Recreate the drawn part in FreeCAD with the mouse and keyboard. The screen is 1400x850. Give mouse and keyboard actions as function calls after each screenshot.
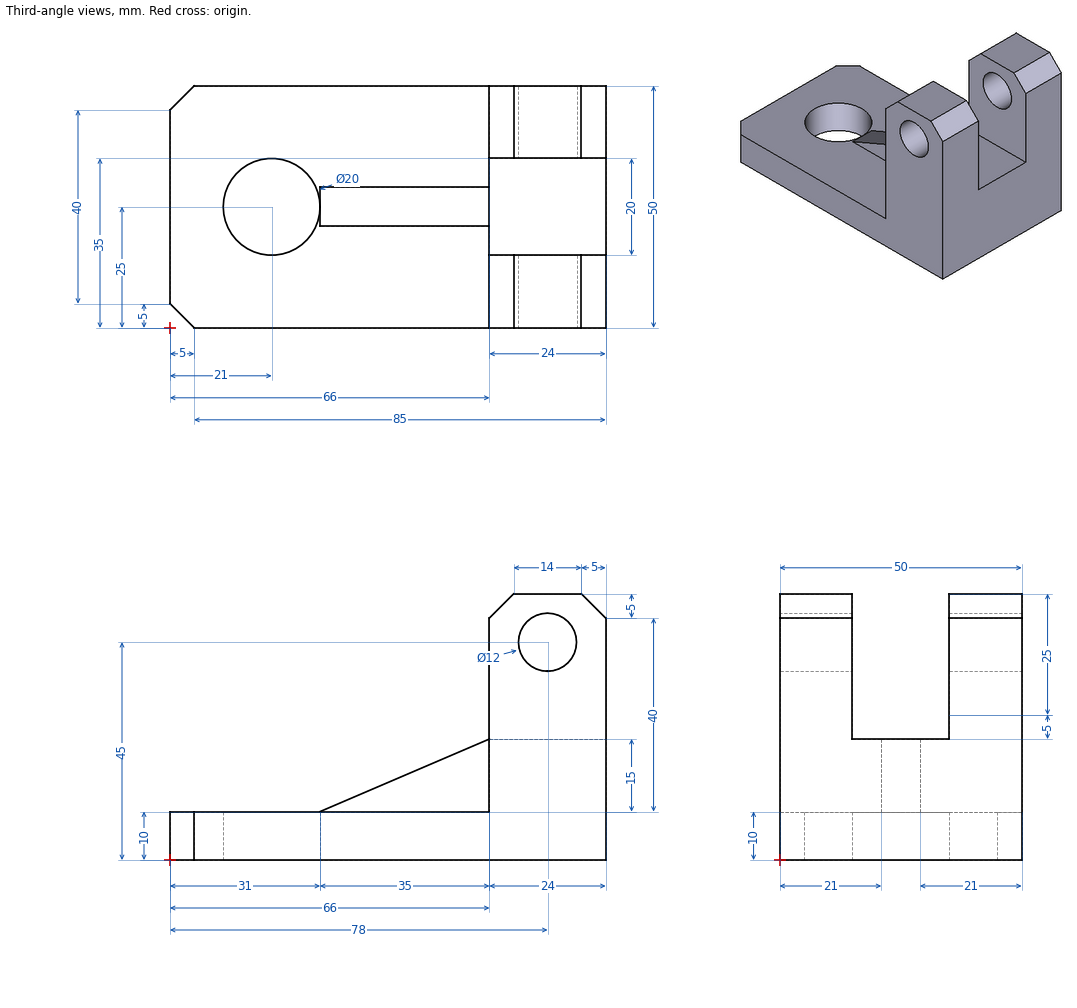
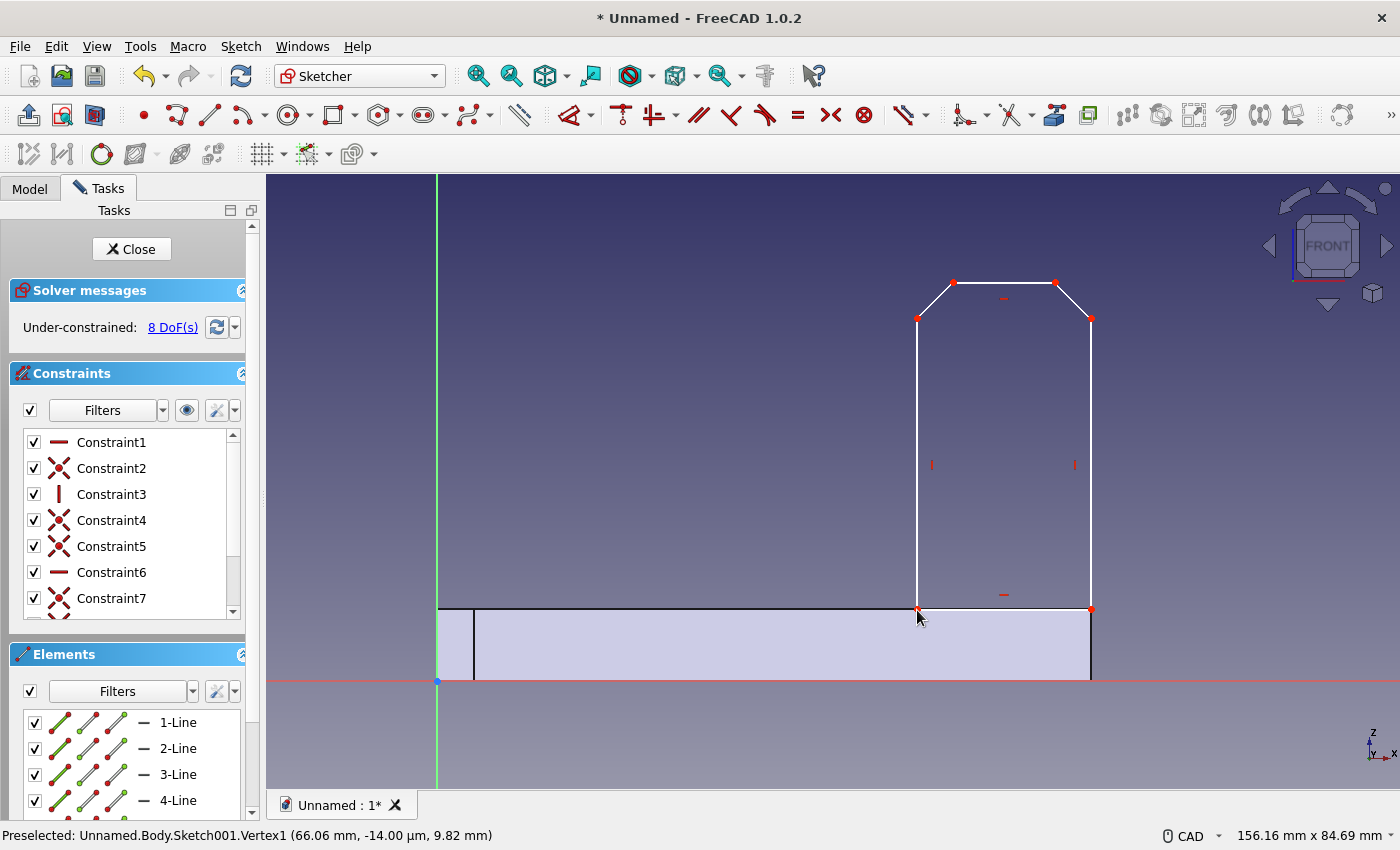
click(568, 116)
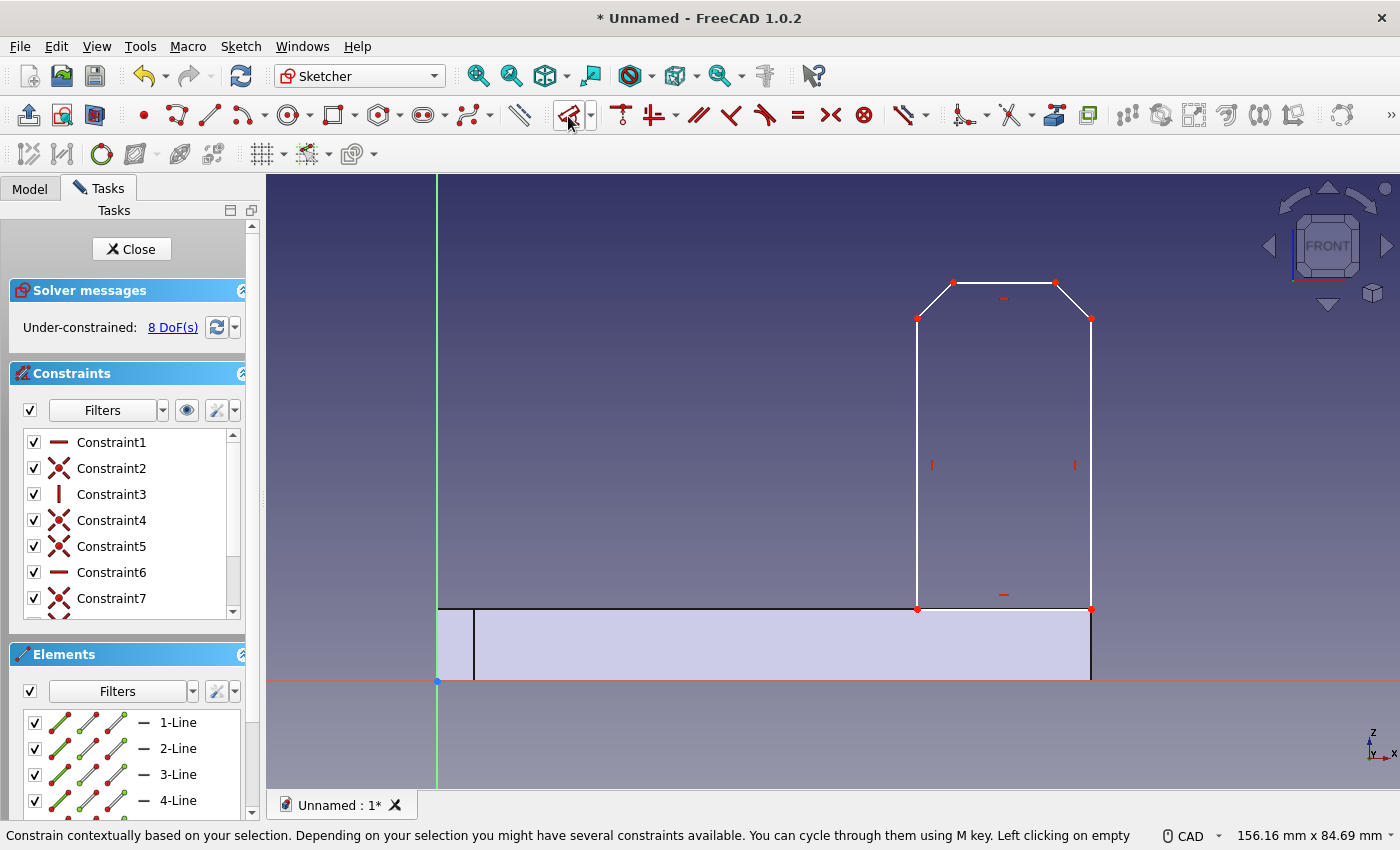
click(969, 610)
click(1004, 644)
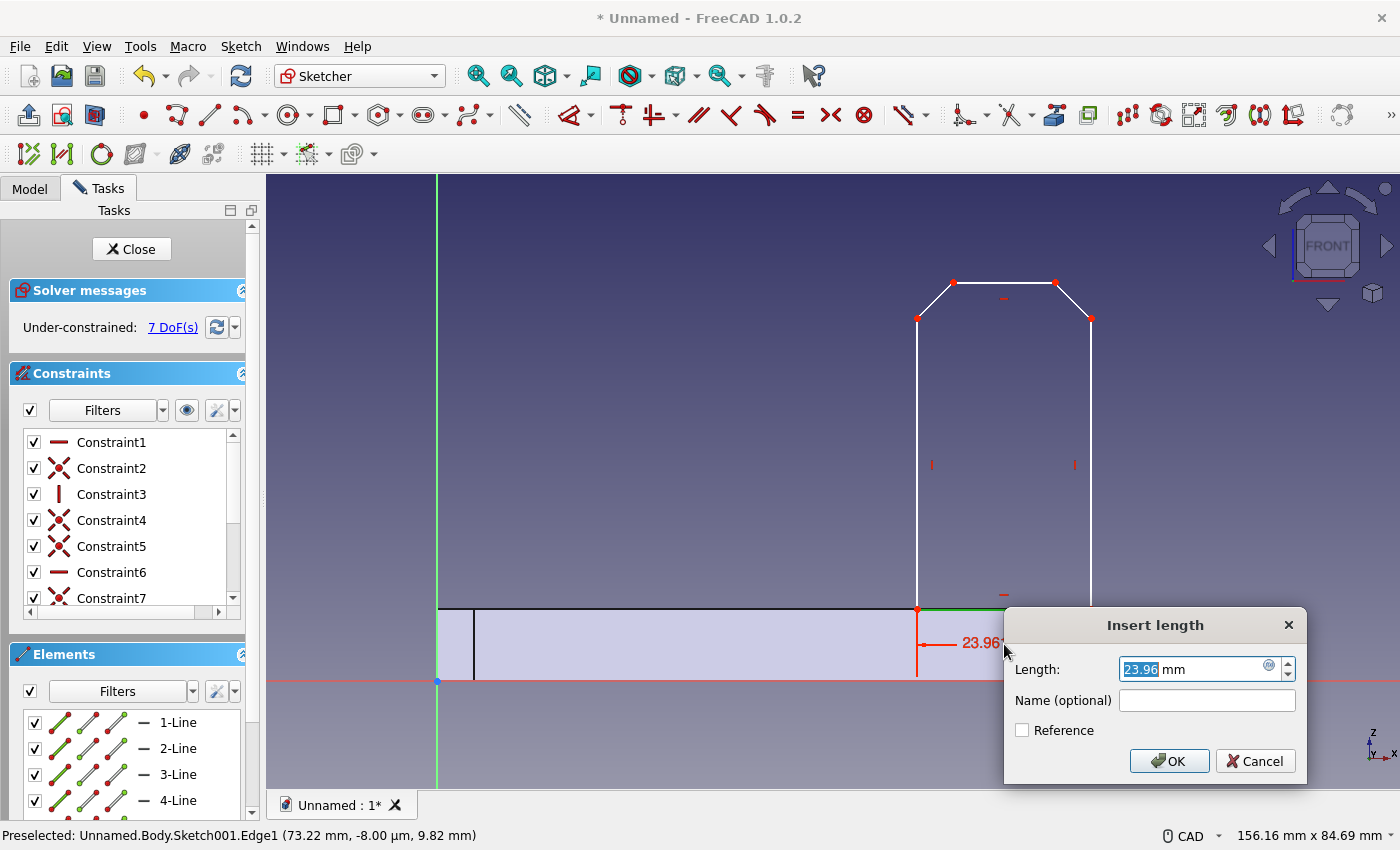
text(24)
key(Return)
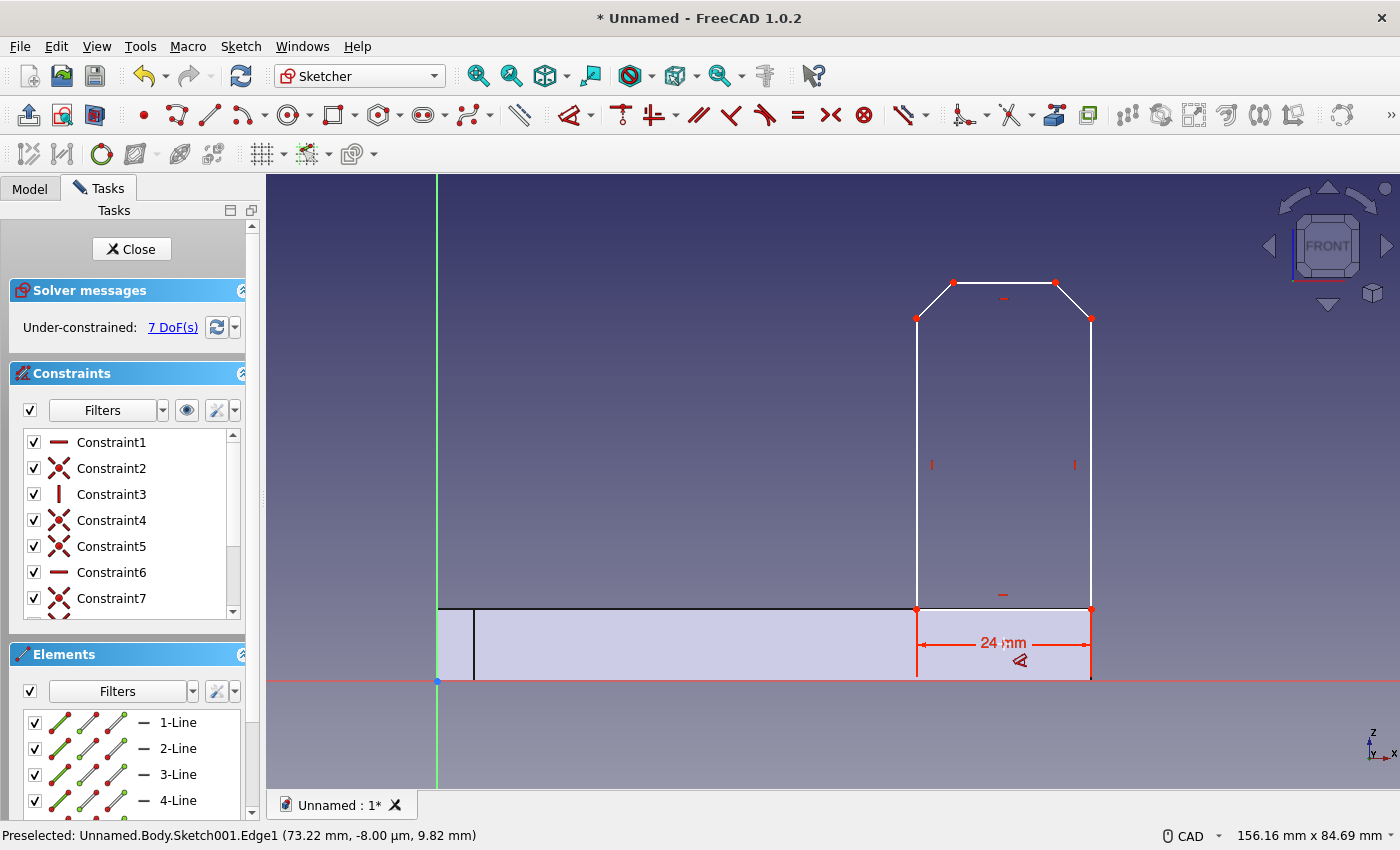
click(1091, 523)
click(1125, 465)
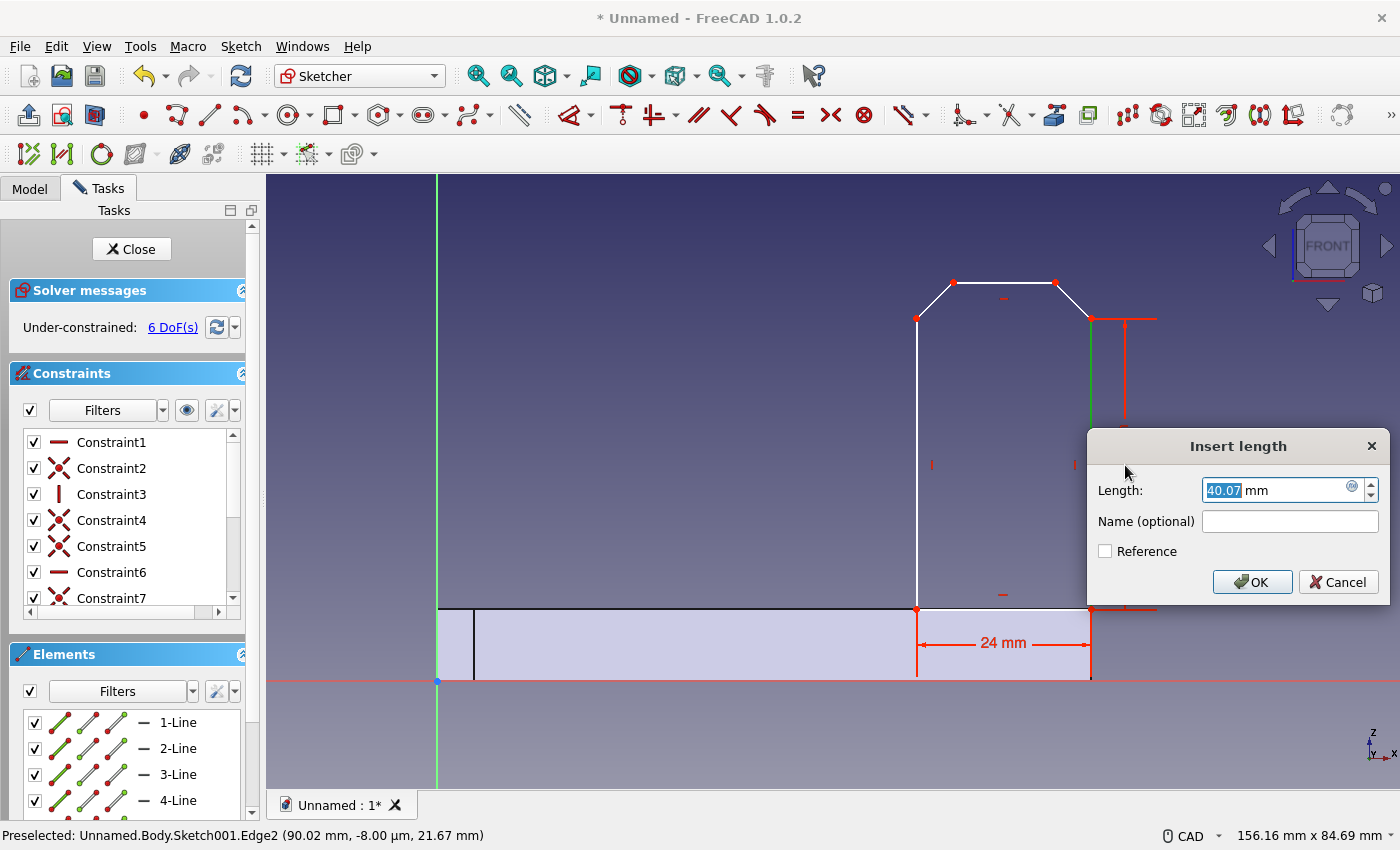
text(40)
key(Return)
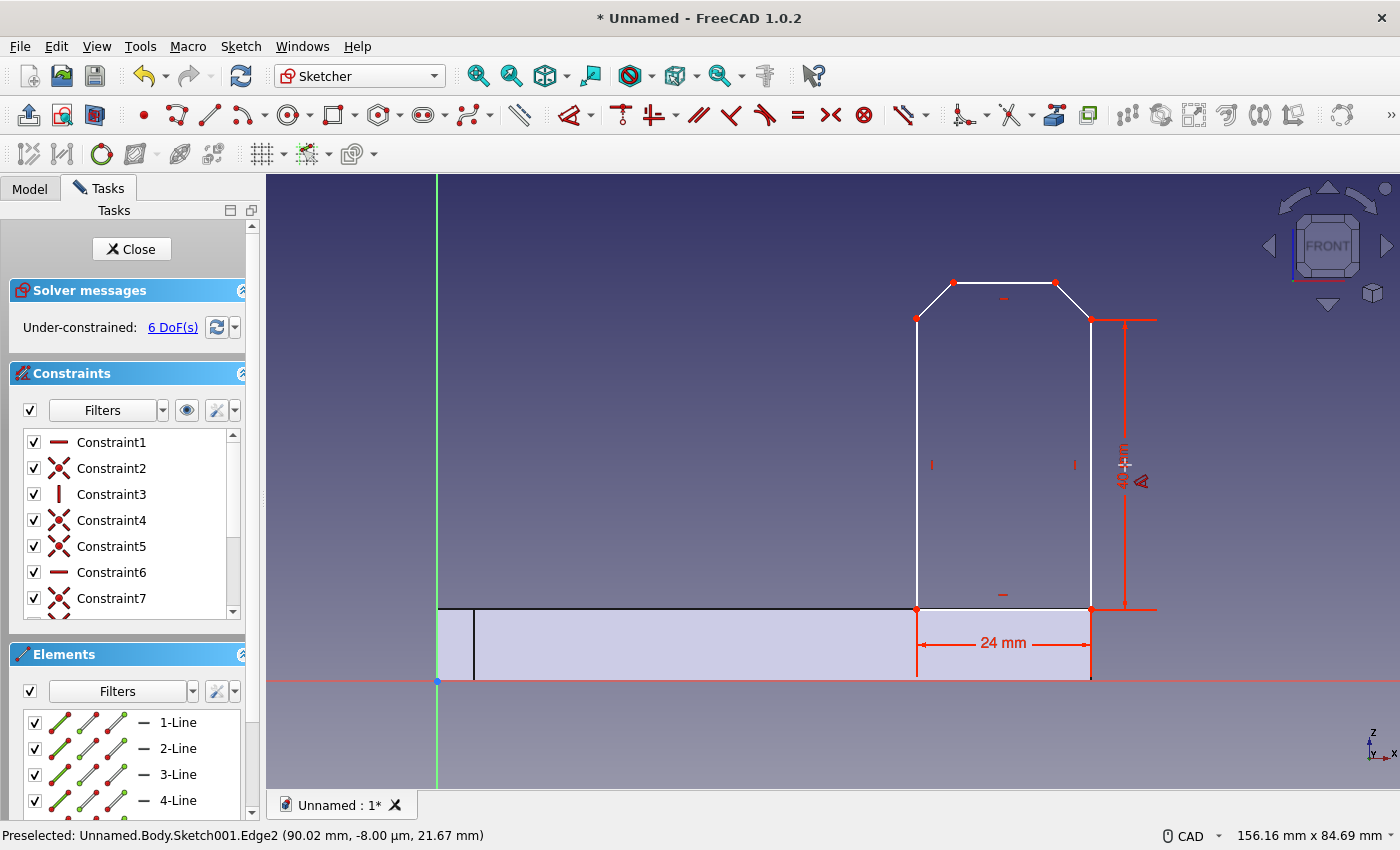
click(1024, 283)
click(1004, 249)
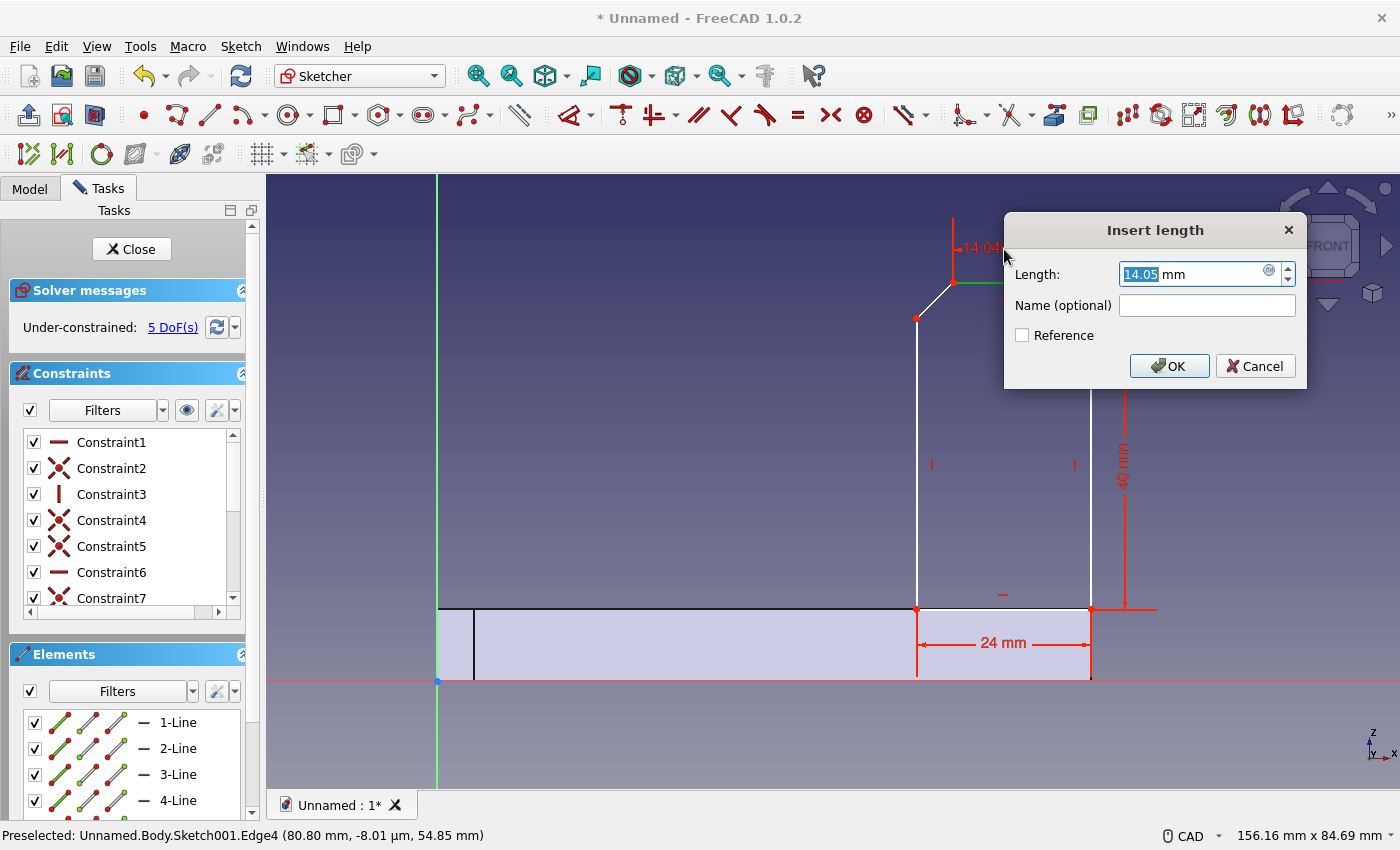
text(14)
key(Return)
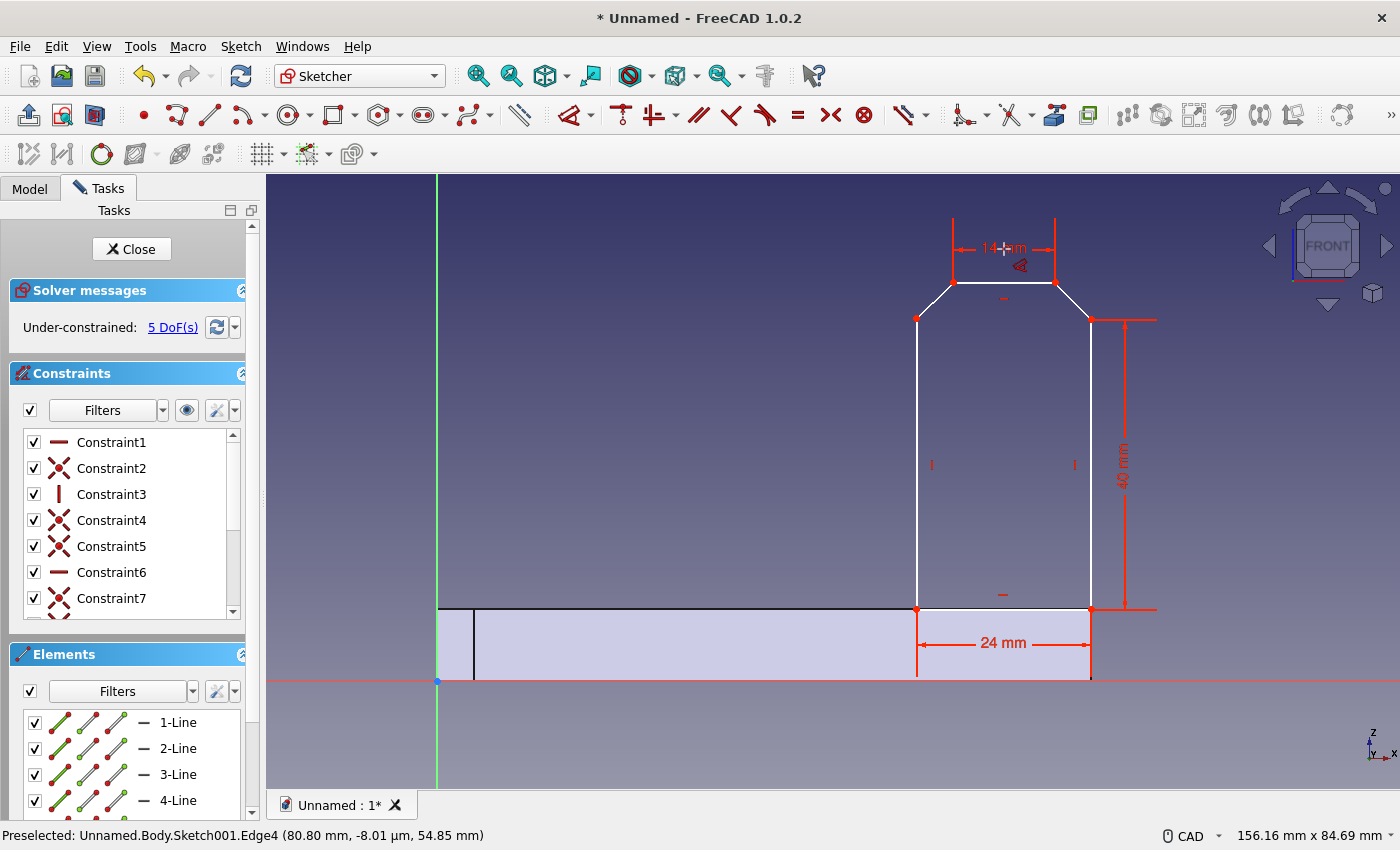
click(917, 406)
click(951, 465)